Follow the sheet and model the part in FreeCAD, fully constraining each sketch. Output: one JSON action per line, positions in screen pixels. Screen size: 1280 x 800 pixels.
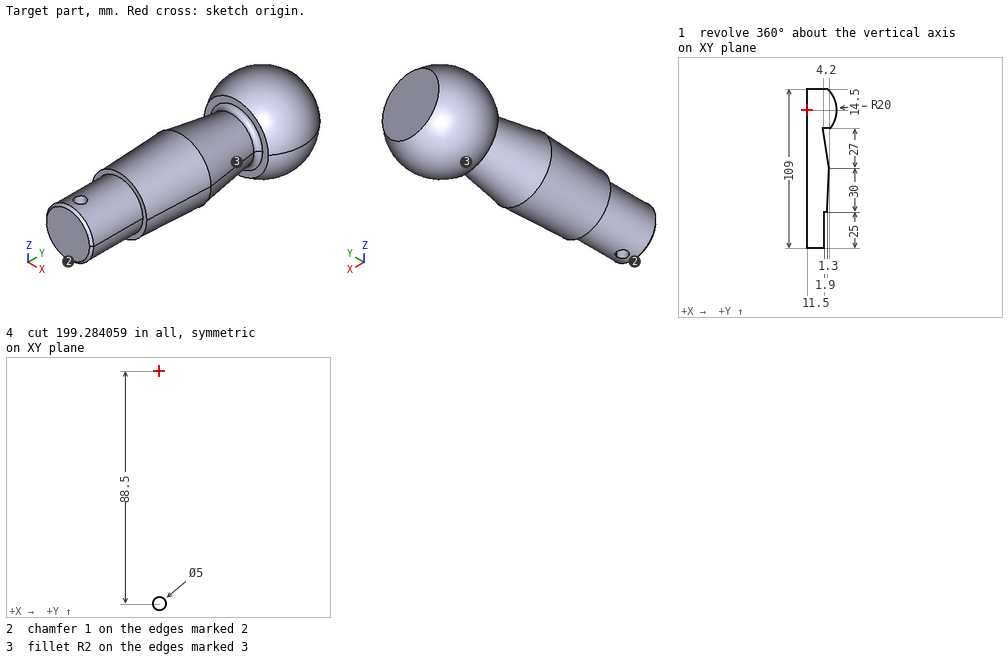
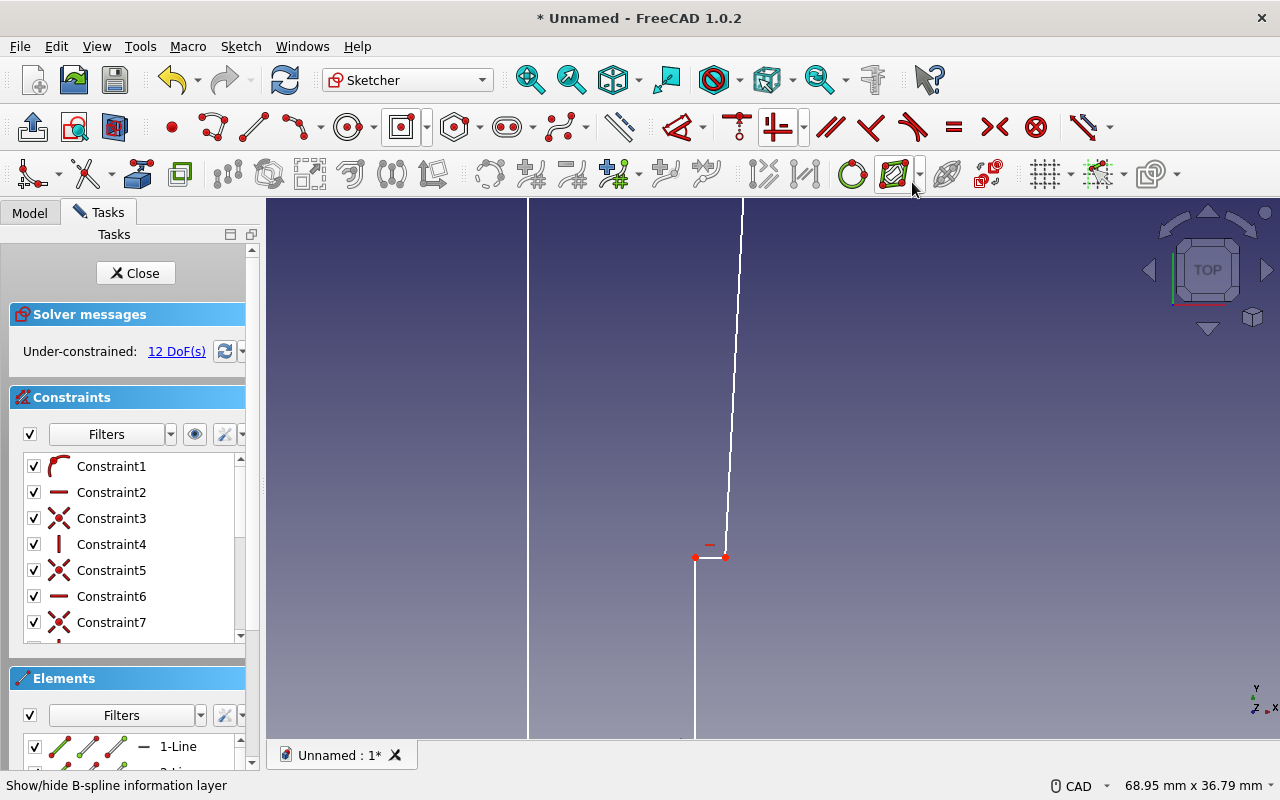
{"action": "scroll", "coordinate": [712, 556], "scroll_direction": "down", "scroll_amount": 8}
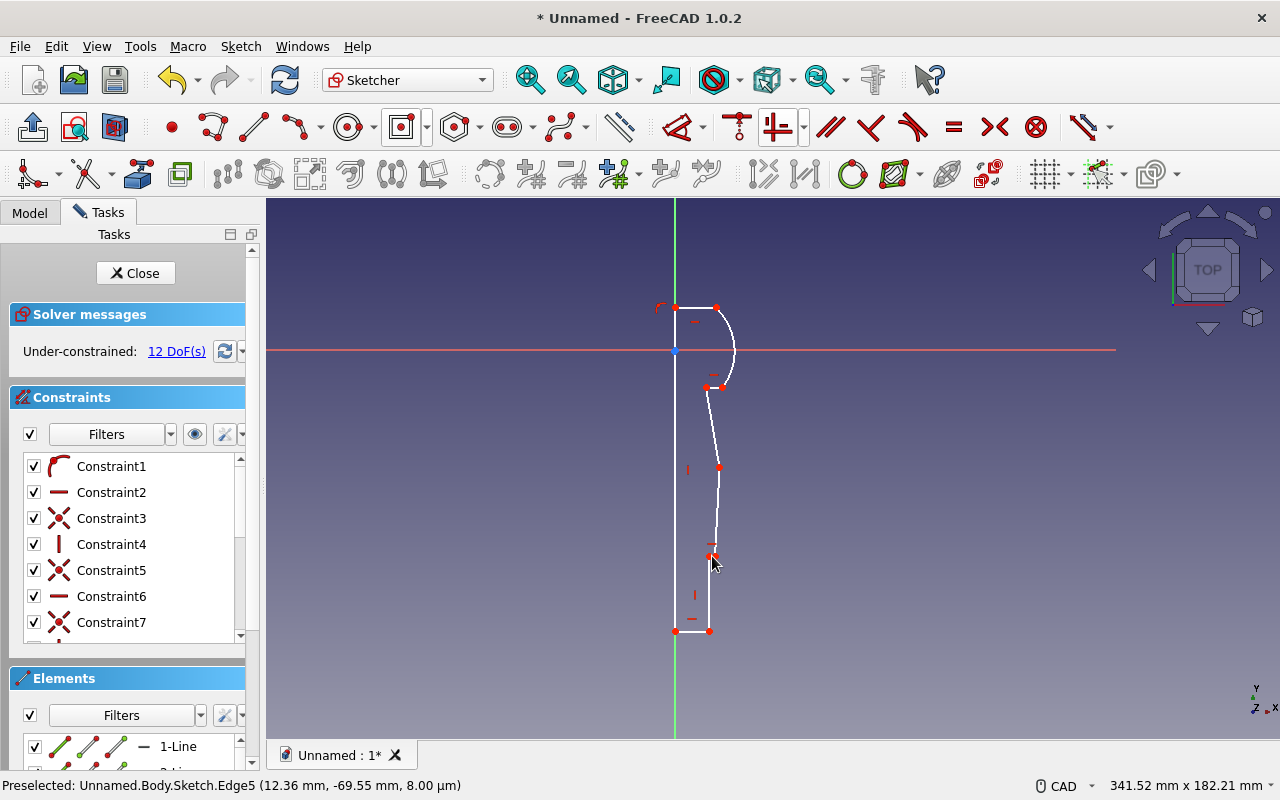
{"action": "left_click_drag", "start_coordinate": [665, 340], "coordinate": [685, 361]}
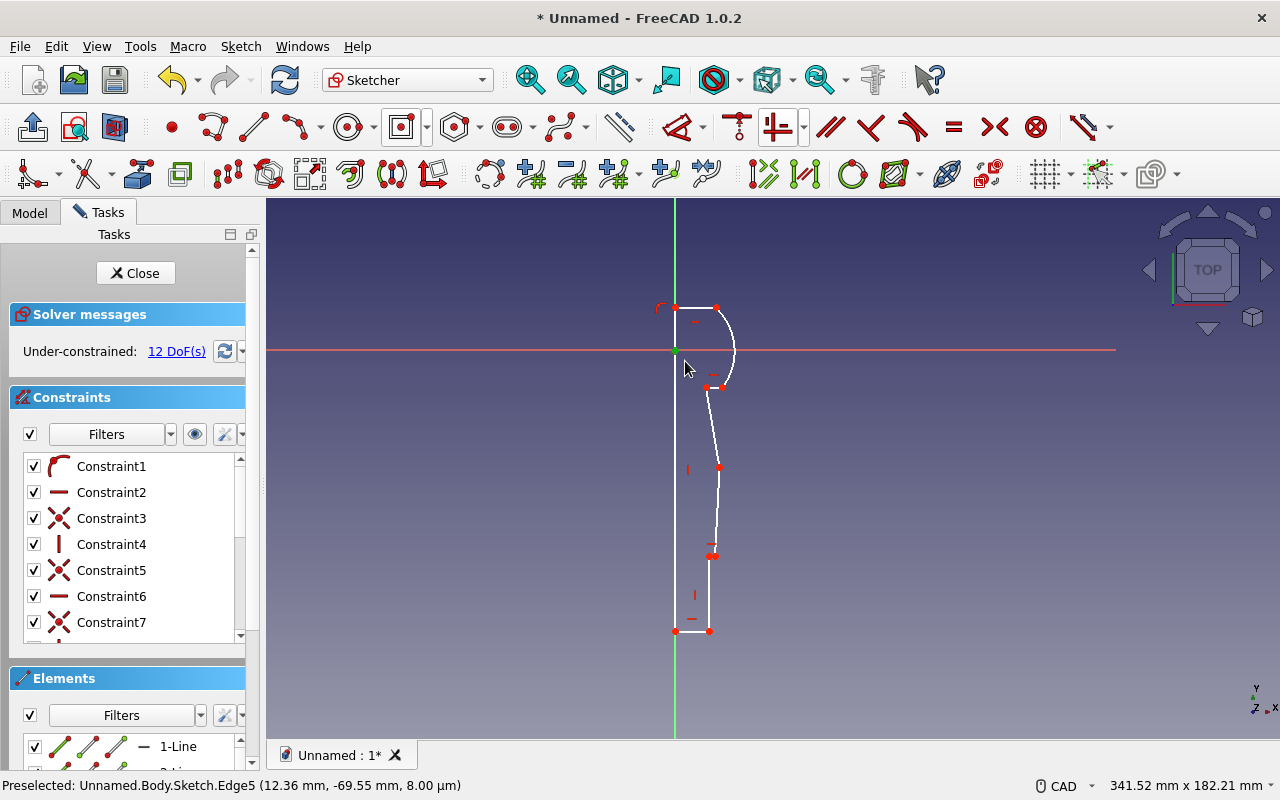
{"action": "left_click", "coordinate": [737, 128]}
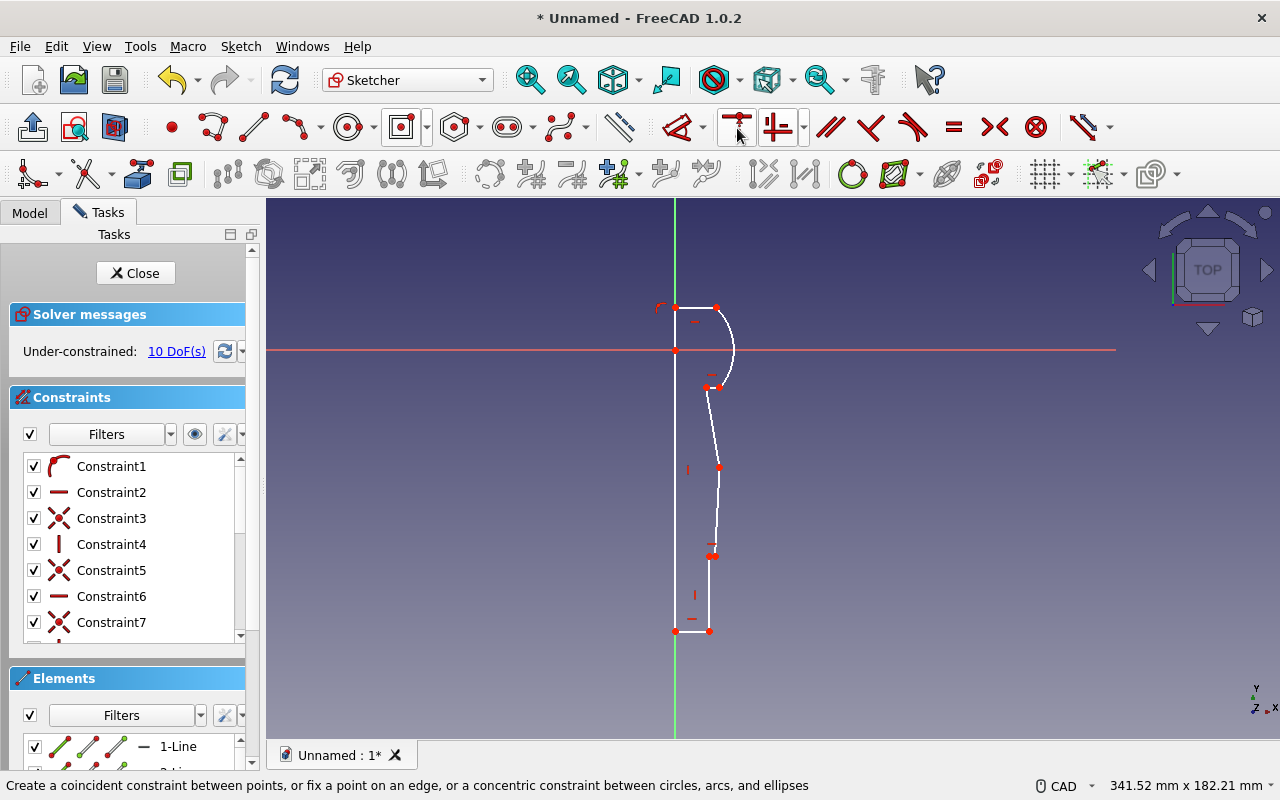
{"action": "left_click", "coordinate": [676, 128]}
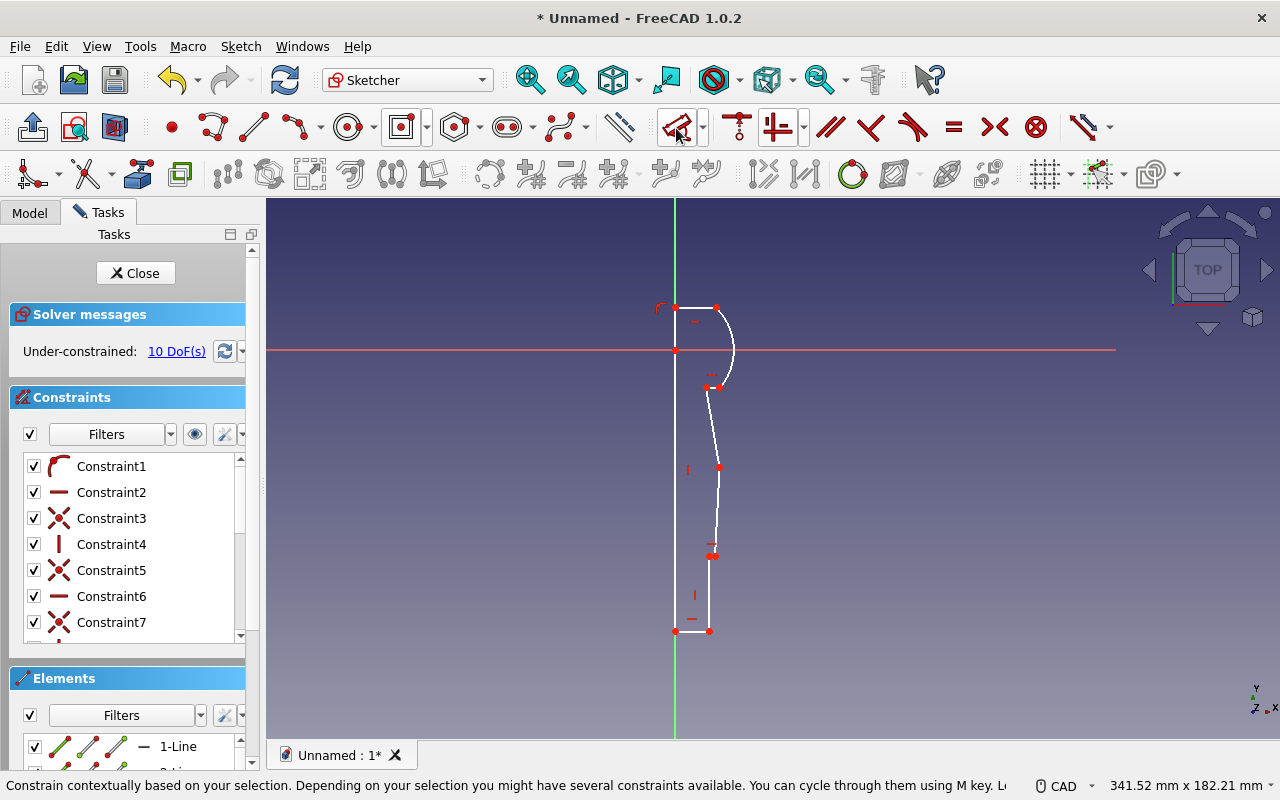
{"action": "left_click", "coordinate": [732, 365]}
{"action": "left_click", "coordinate": [763, 373]}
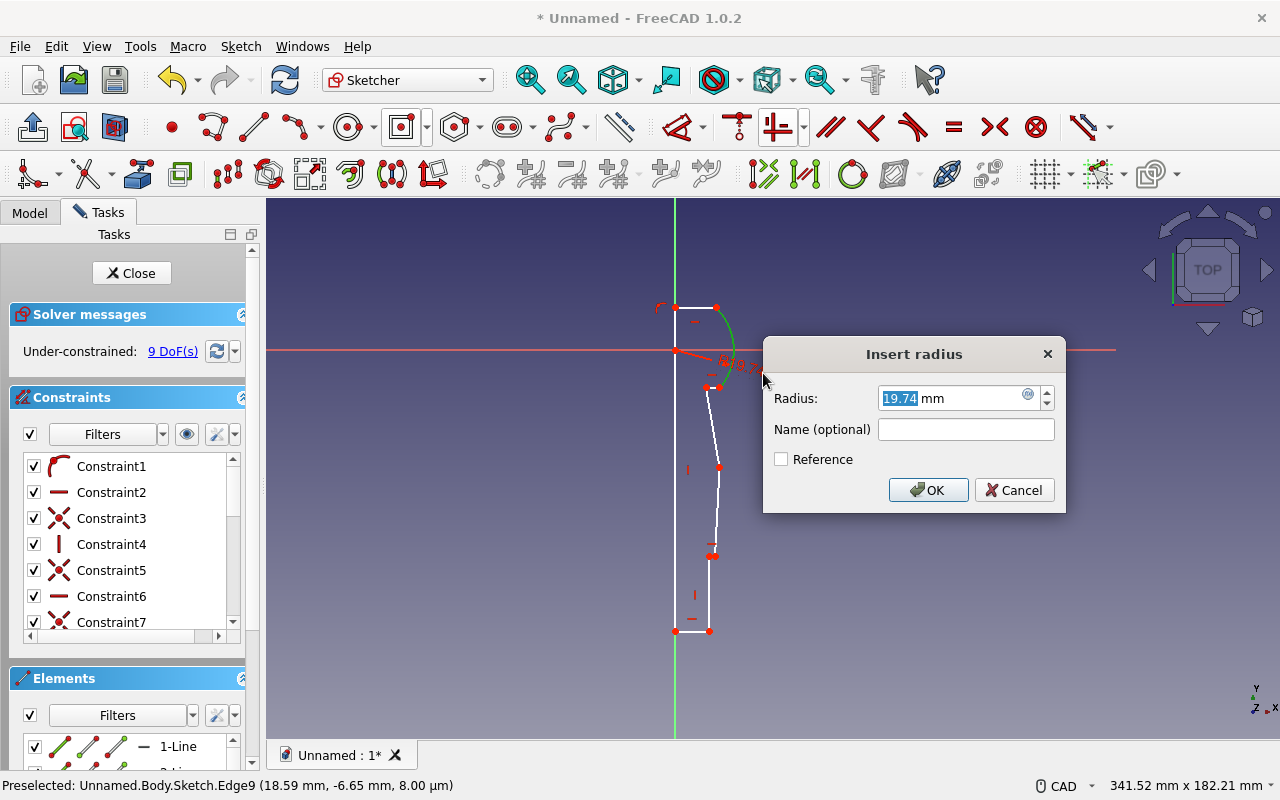
{"action": "type", "text": "20"}
{"action": "key", "text": "Return"}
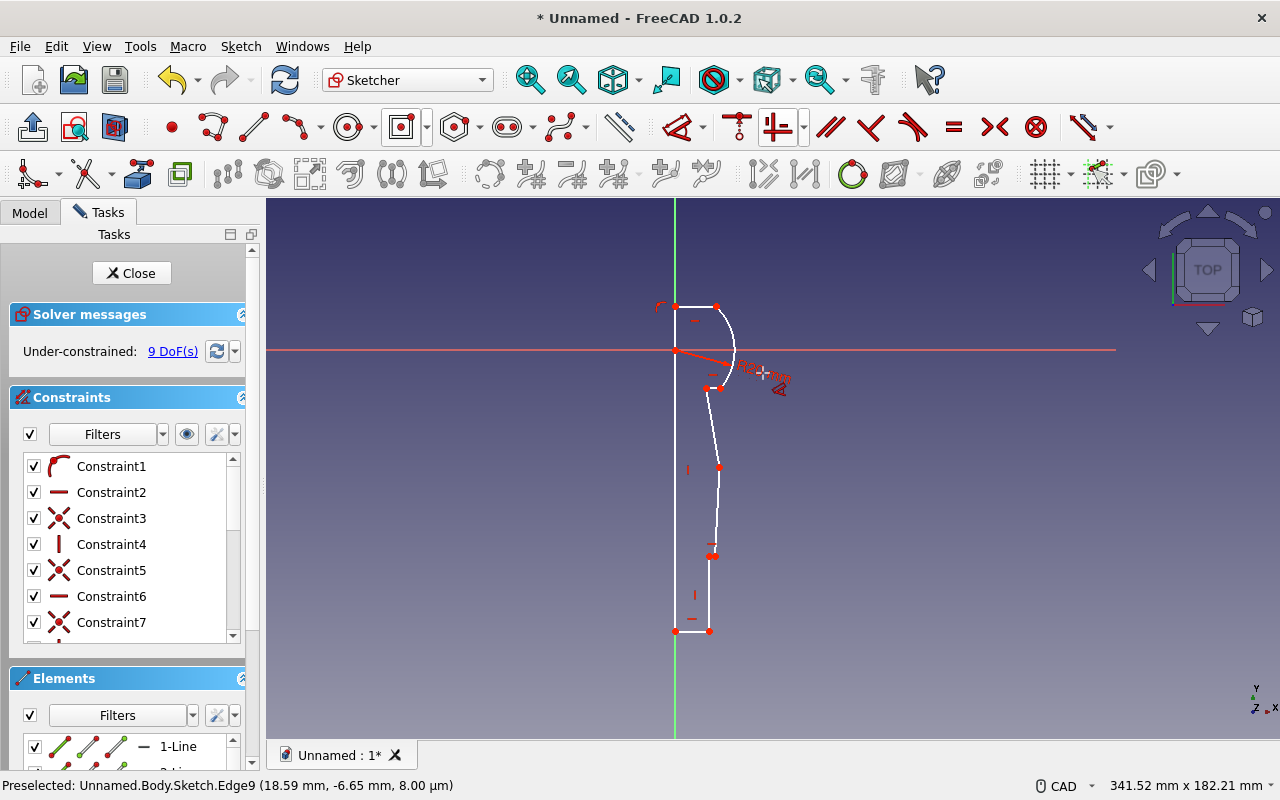
{"action": "left_click", "coordinate": [709, 609]}
{"action": "left_click", "coordinate": [743, 594]}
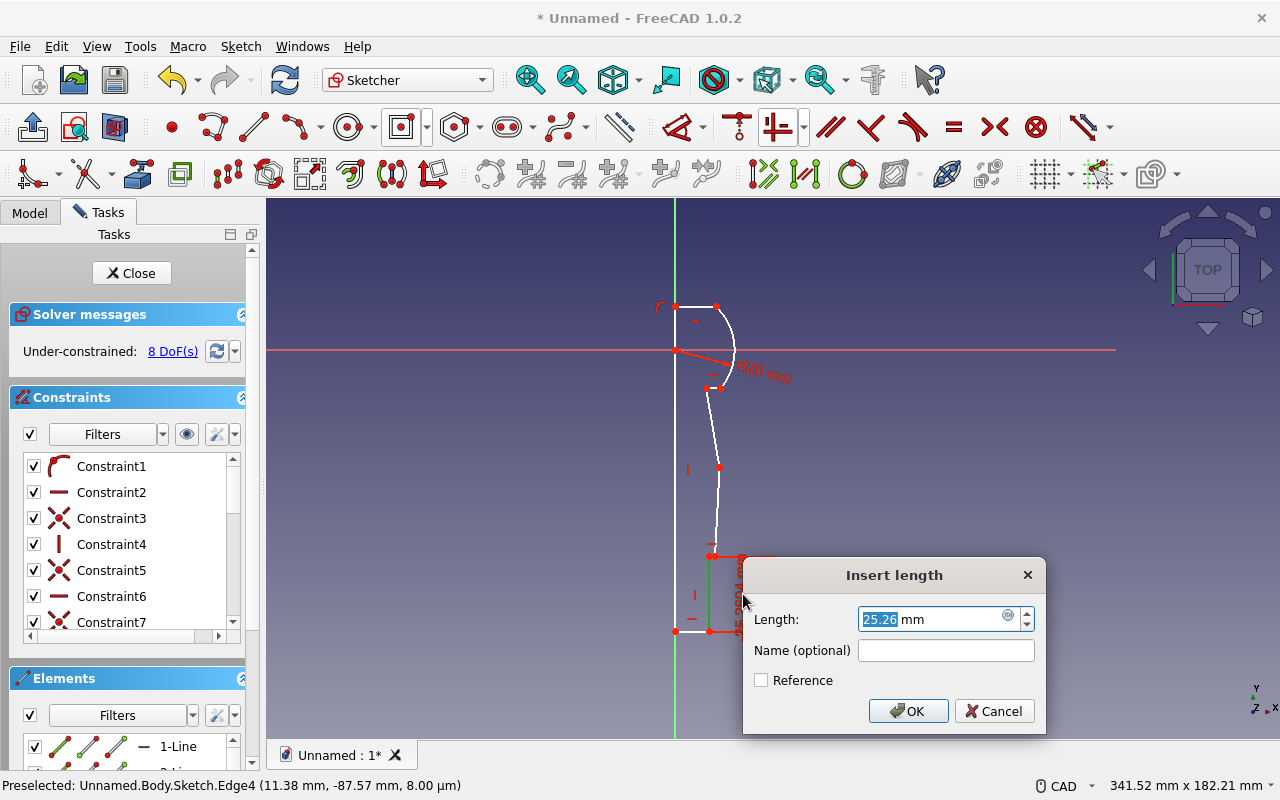
{"action": "type", "text": "25"}
{"action": "key", "text": "Return"}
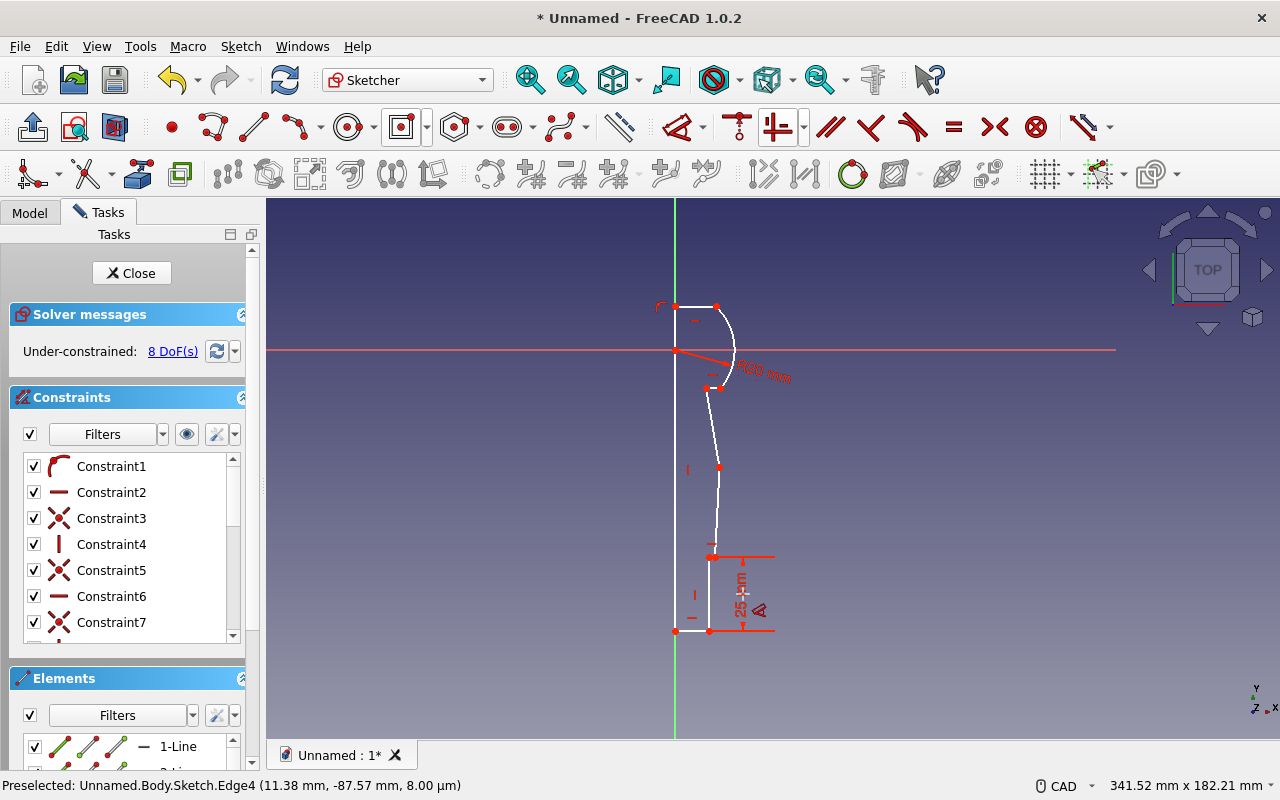
{"action": "left_click", "coordinate": [675, 404]}
{"action": "left_click", "coordinate": [641, 469]}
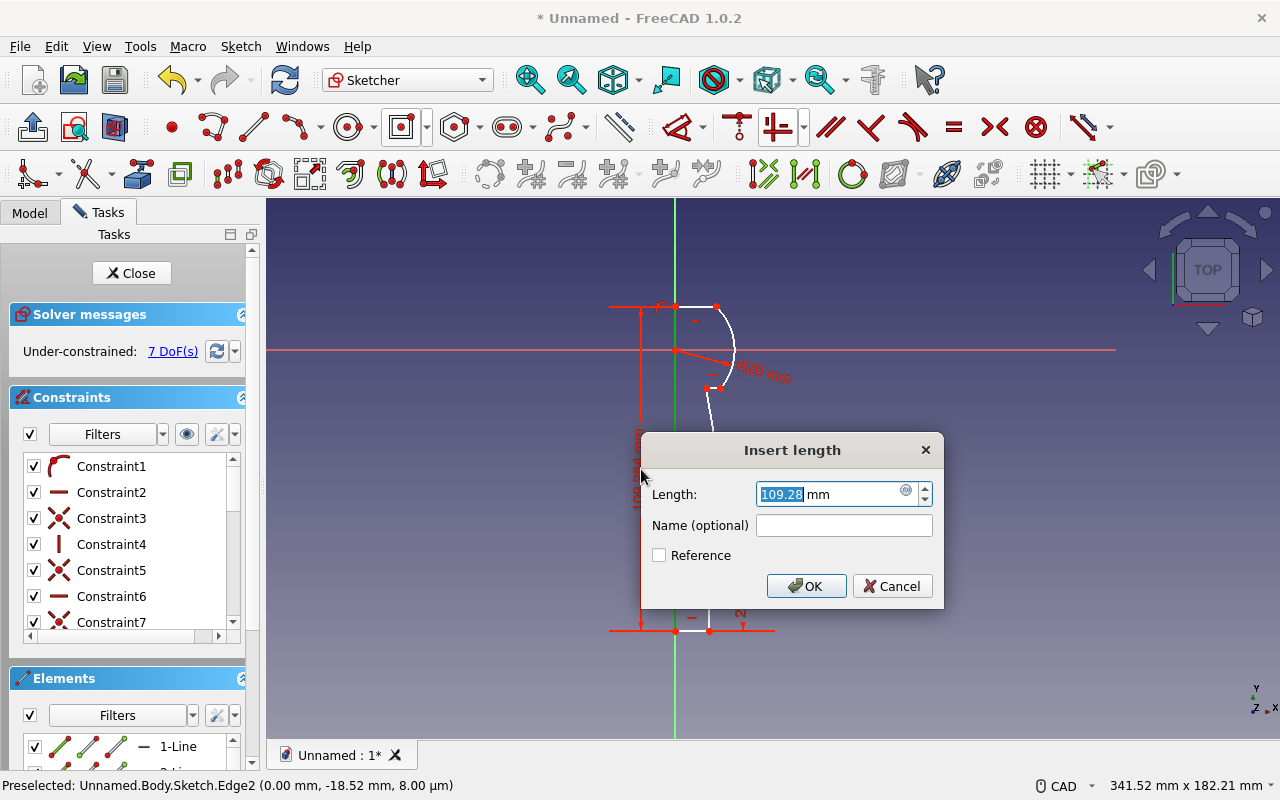
{"action": "type", "text": "109"}
{"action": "key", "text": "Return"}